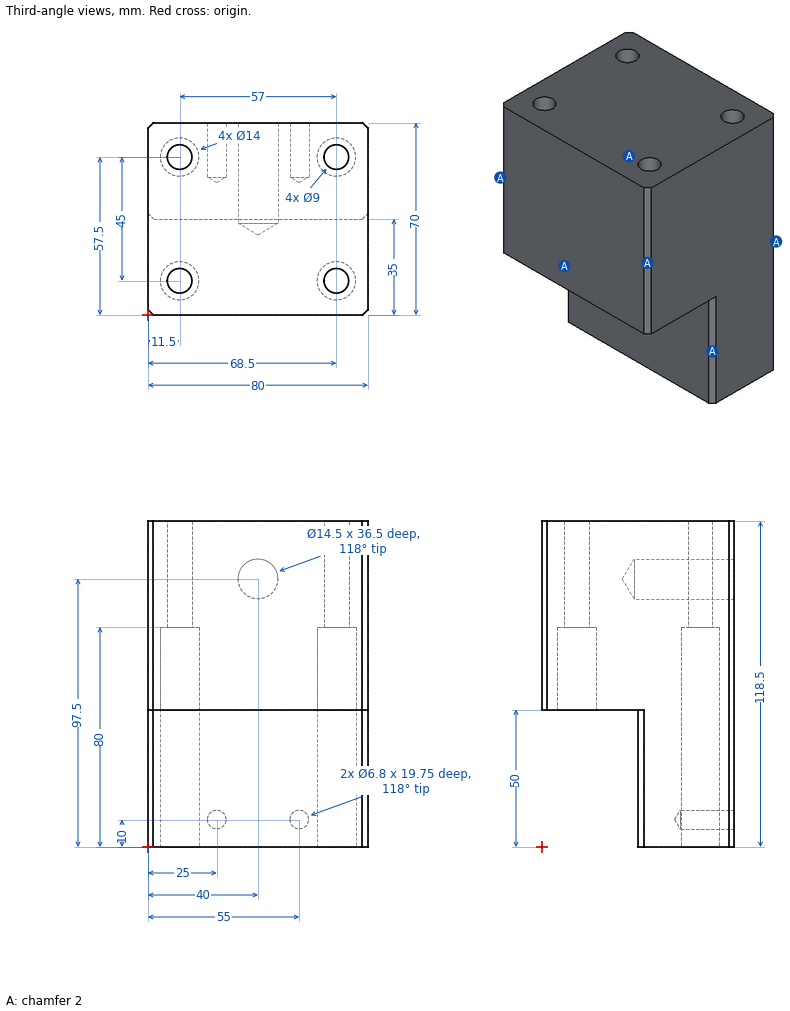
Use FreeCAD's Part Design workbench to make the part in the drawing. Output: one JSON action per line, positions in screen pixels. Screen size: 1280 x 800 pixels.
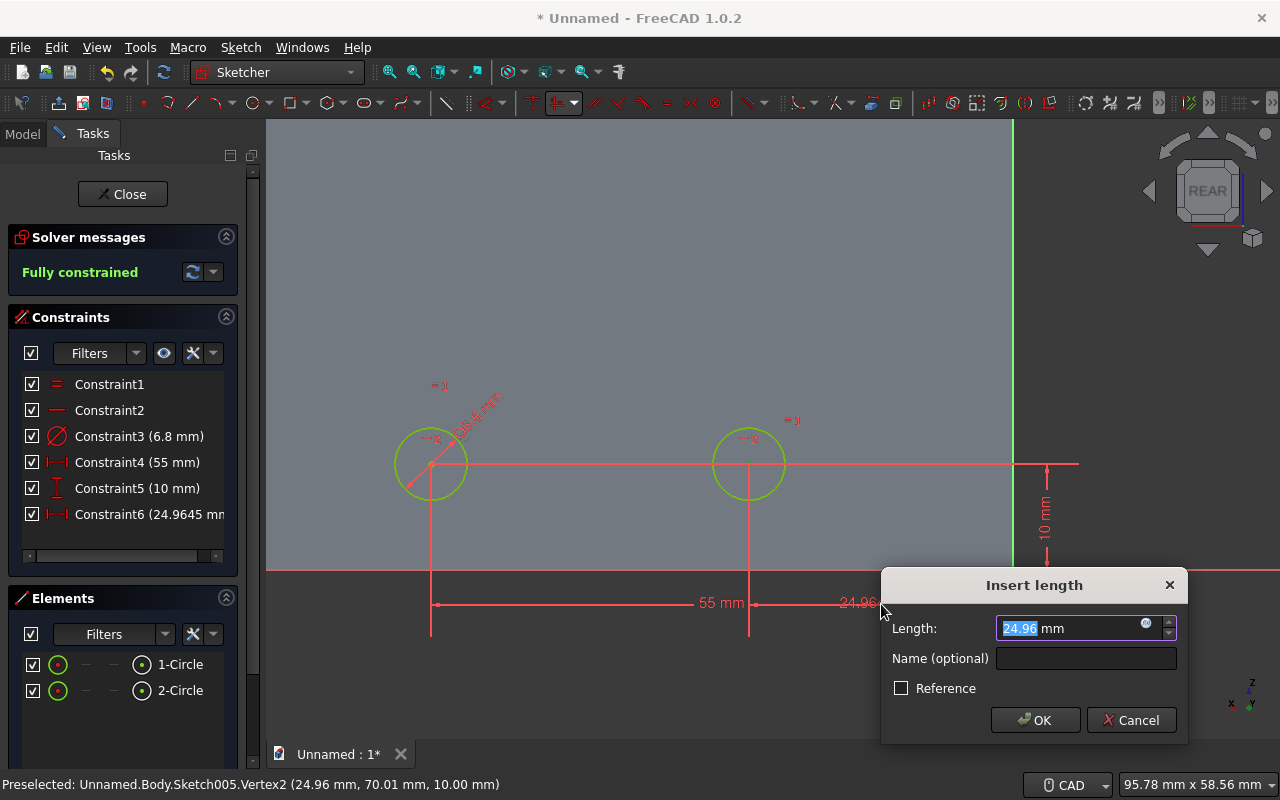
{"action": "type", "text": "25"}
{"action": "key", "text": "Return"}
{"action": "key", "text": "Escape"}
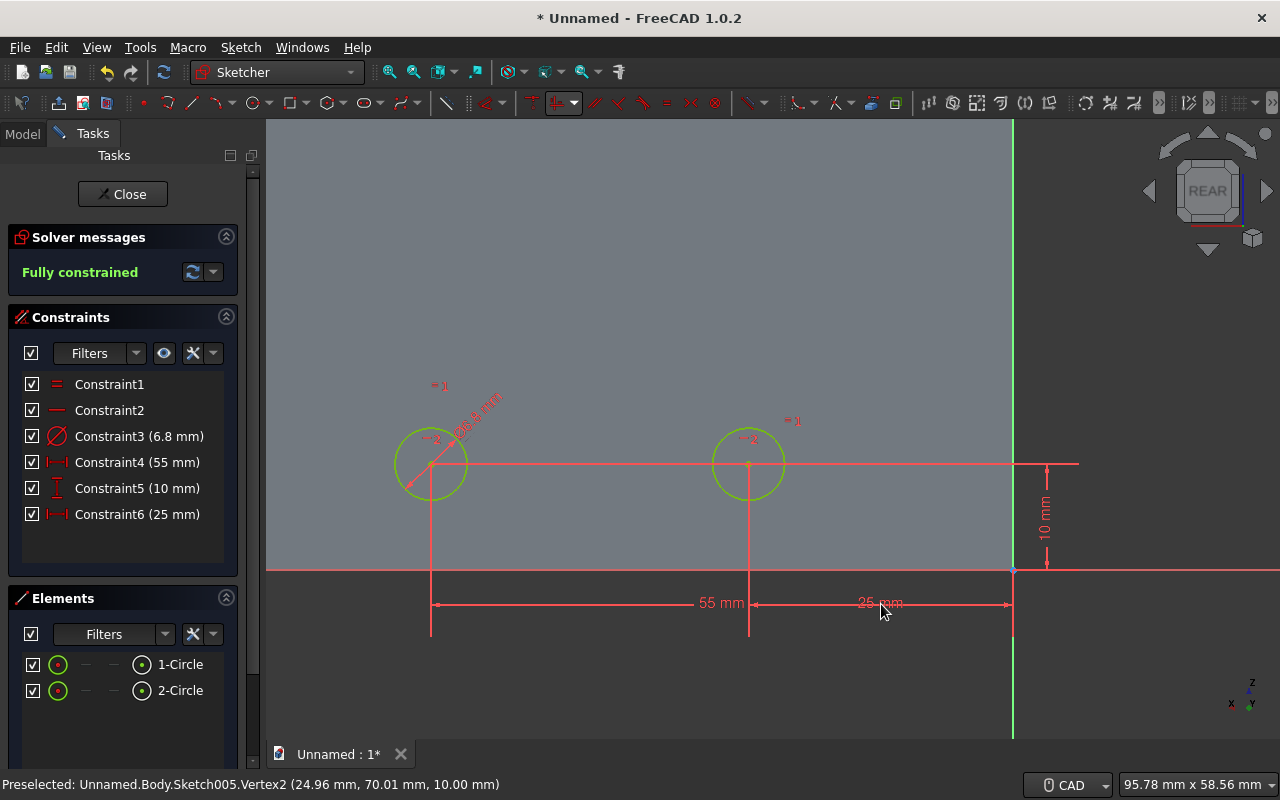
{"action": "left_click", "coordinate": [123, 194]}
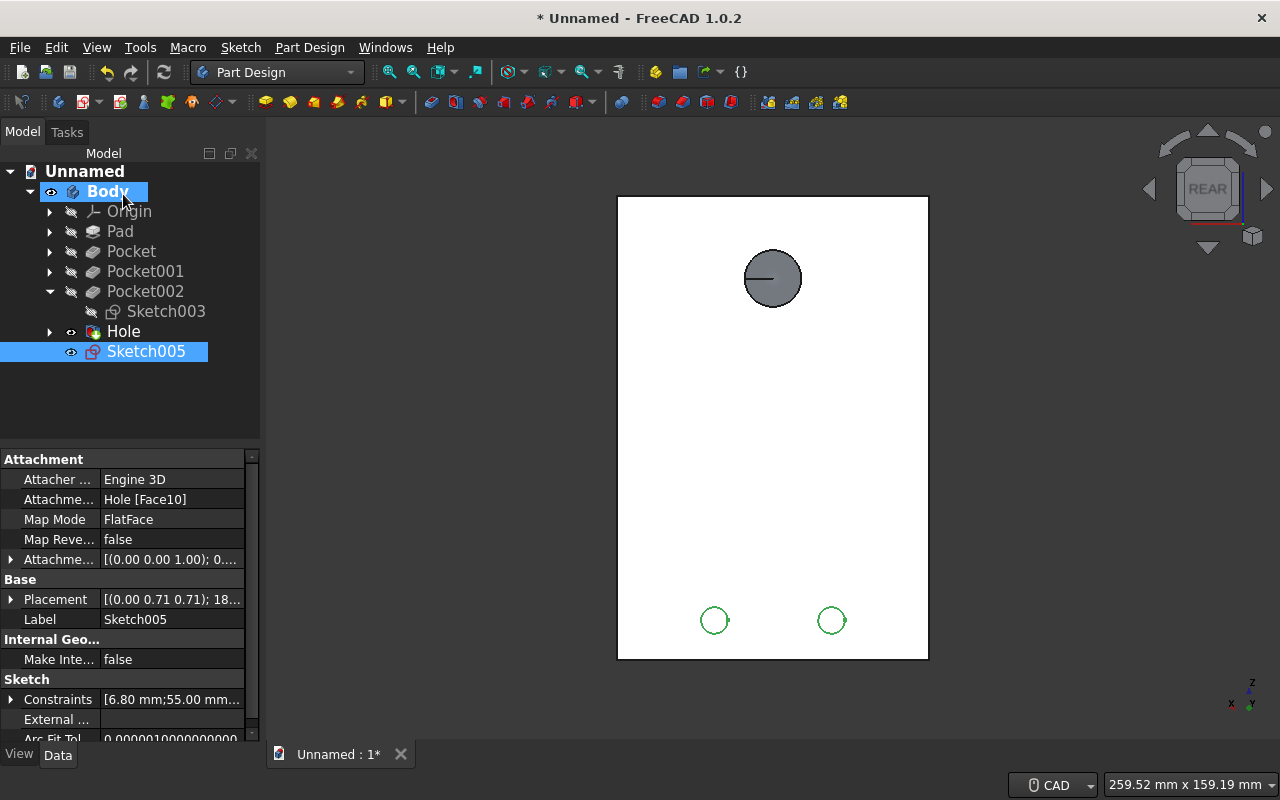
{"action": "left_click", "coordinate": [456, 102]}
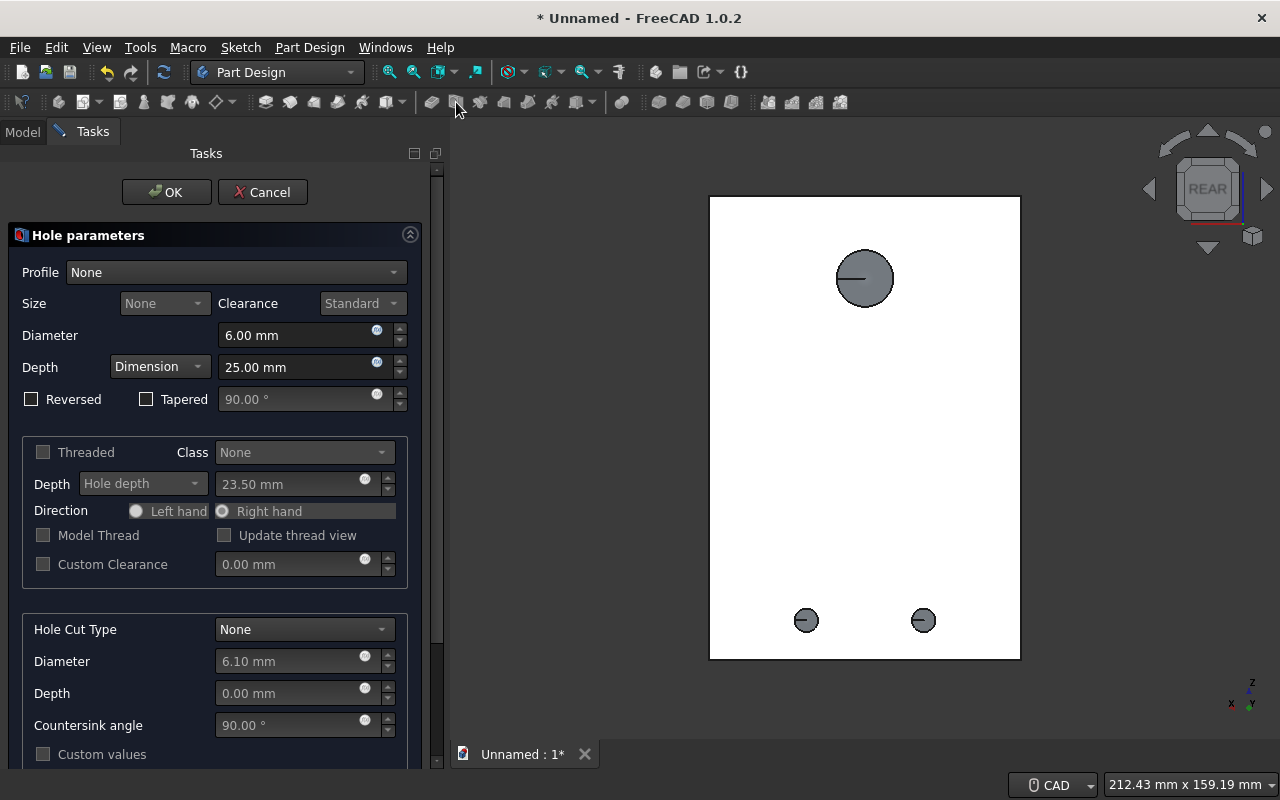
{"action": "triple_click", "coordinate": [305, 335]}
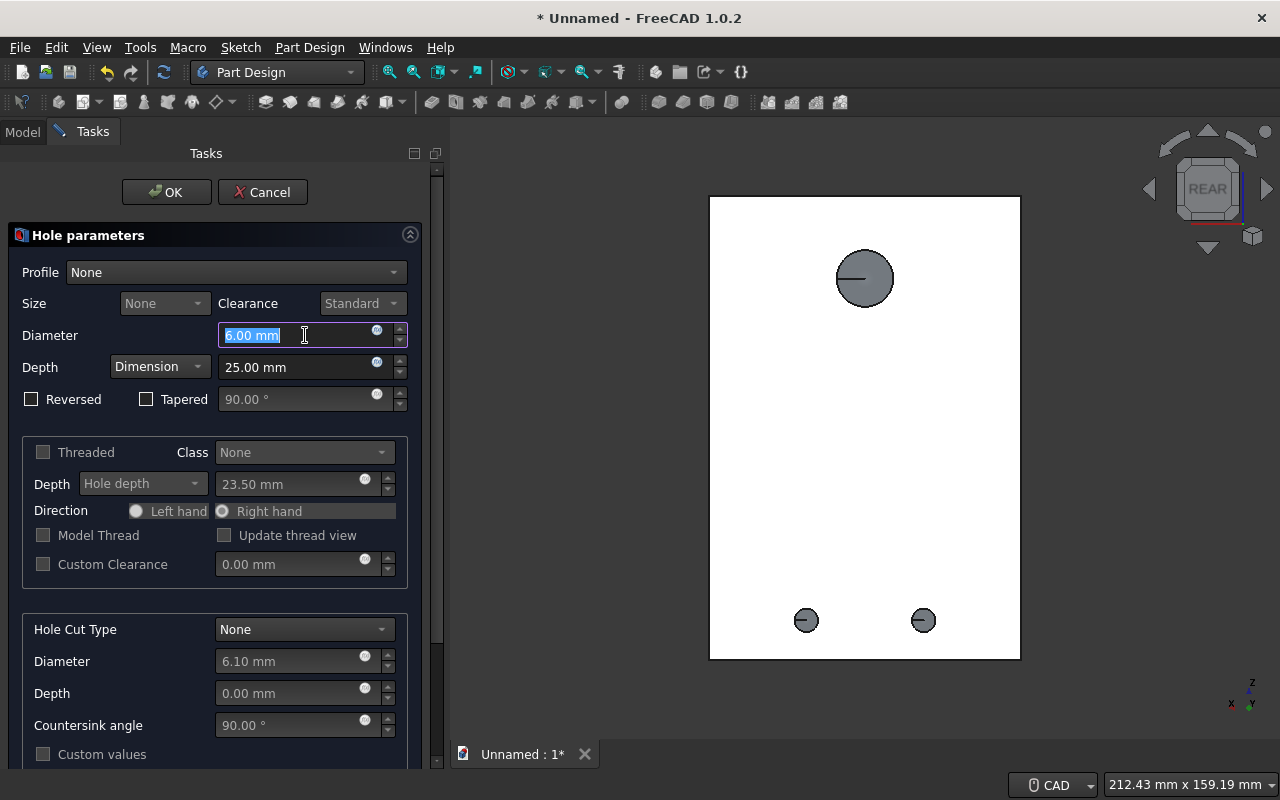
{"action": "type", "text": "6.8"}
{"action": "key", "text": "Tab"}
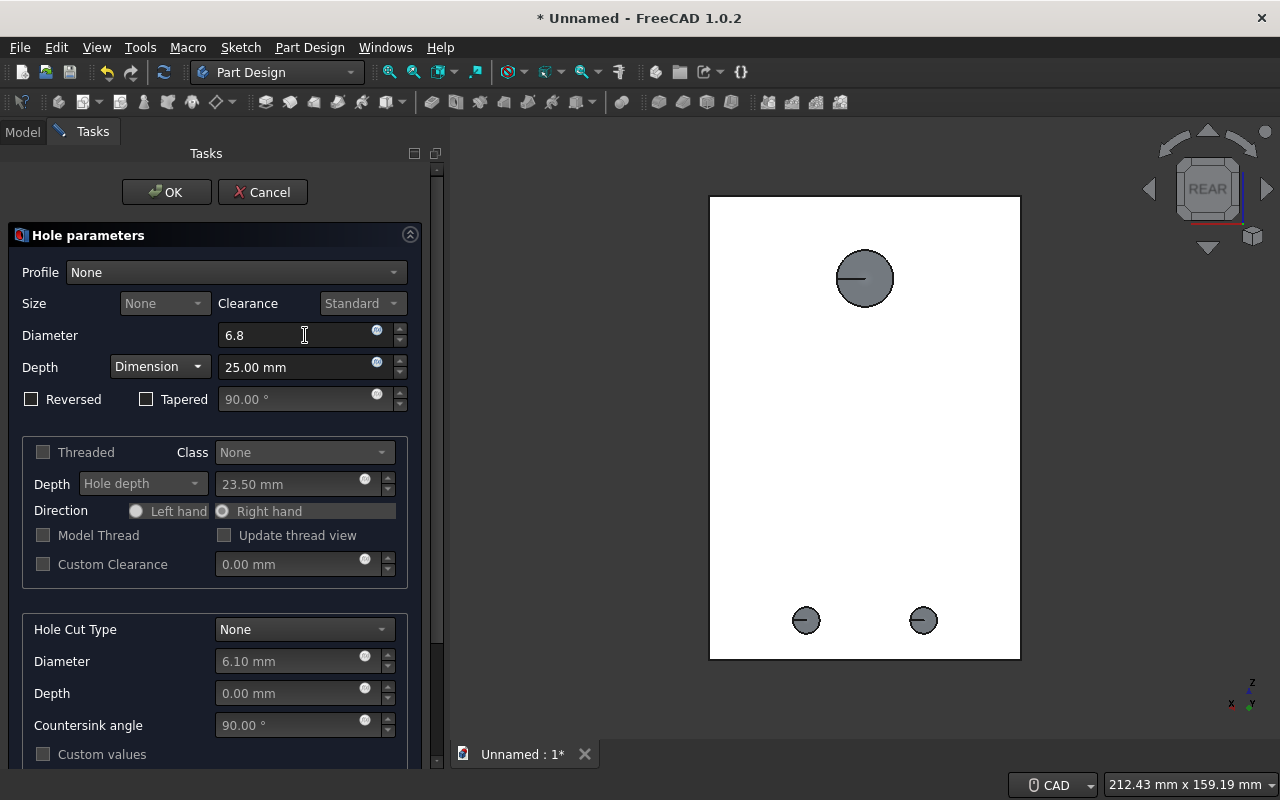
{"action": "triple_click", "coordinate": [305, 367]}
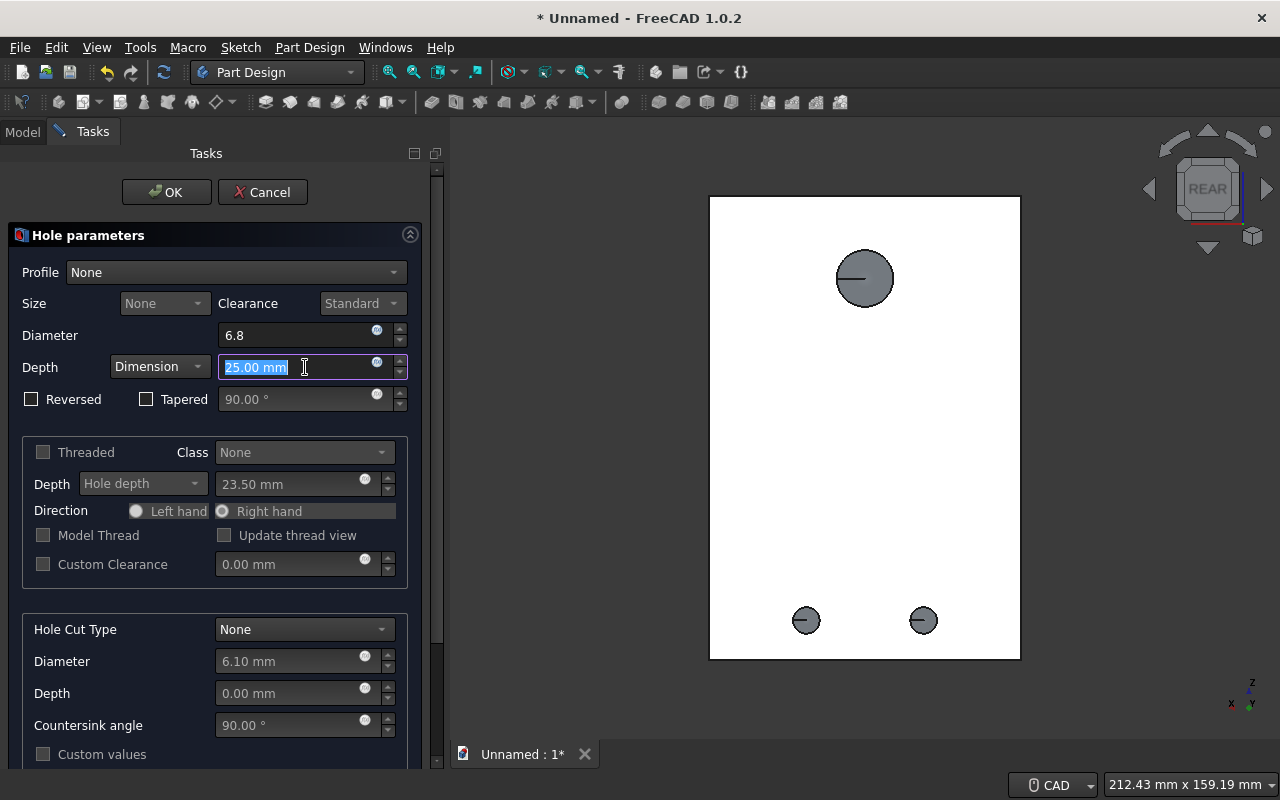
{"action": "type", "text": "19.75"}
{"action": "key", "text": "Tab"}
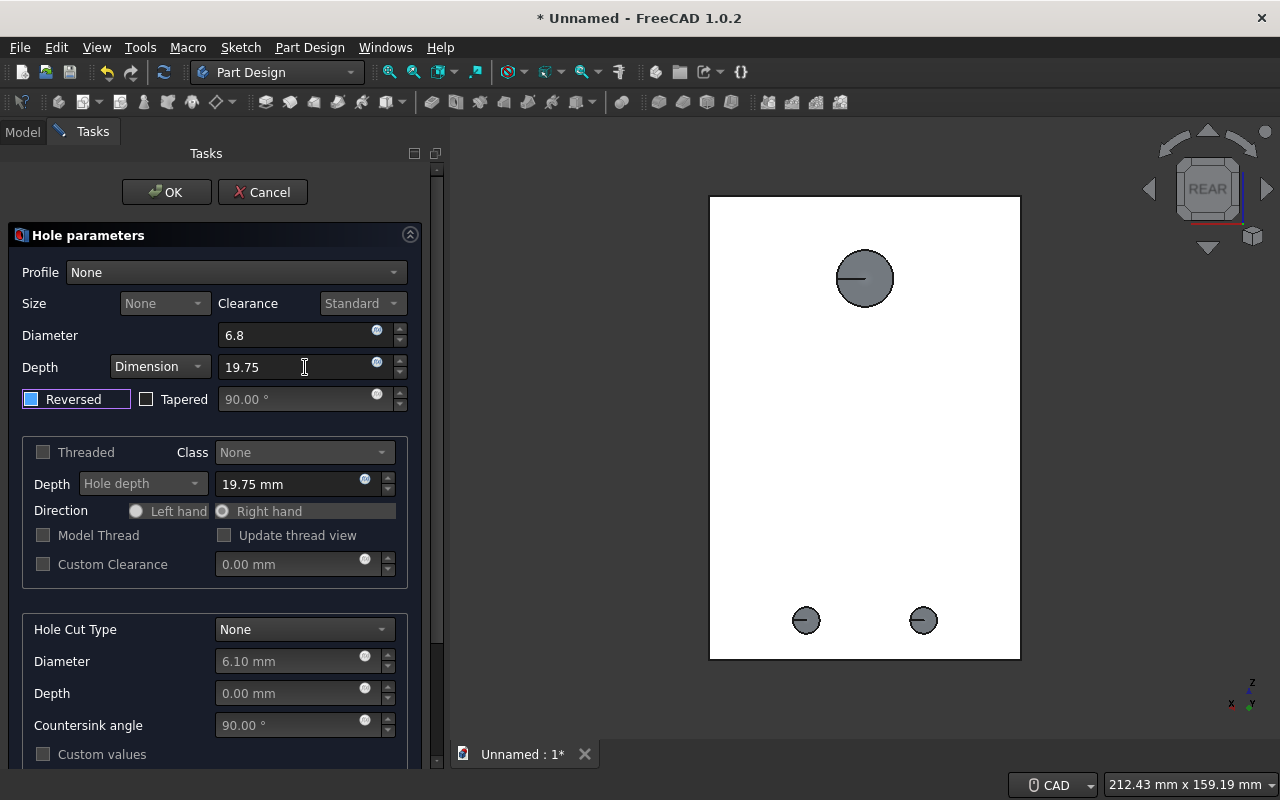
{"action": "left_click", "coordinate": [167, 192]}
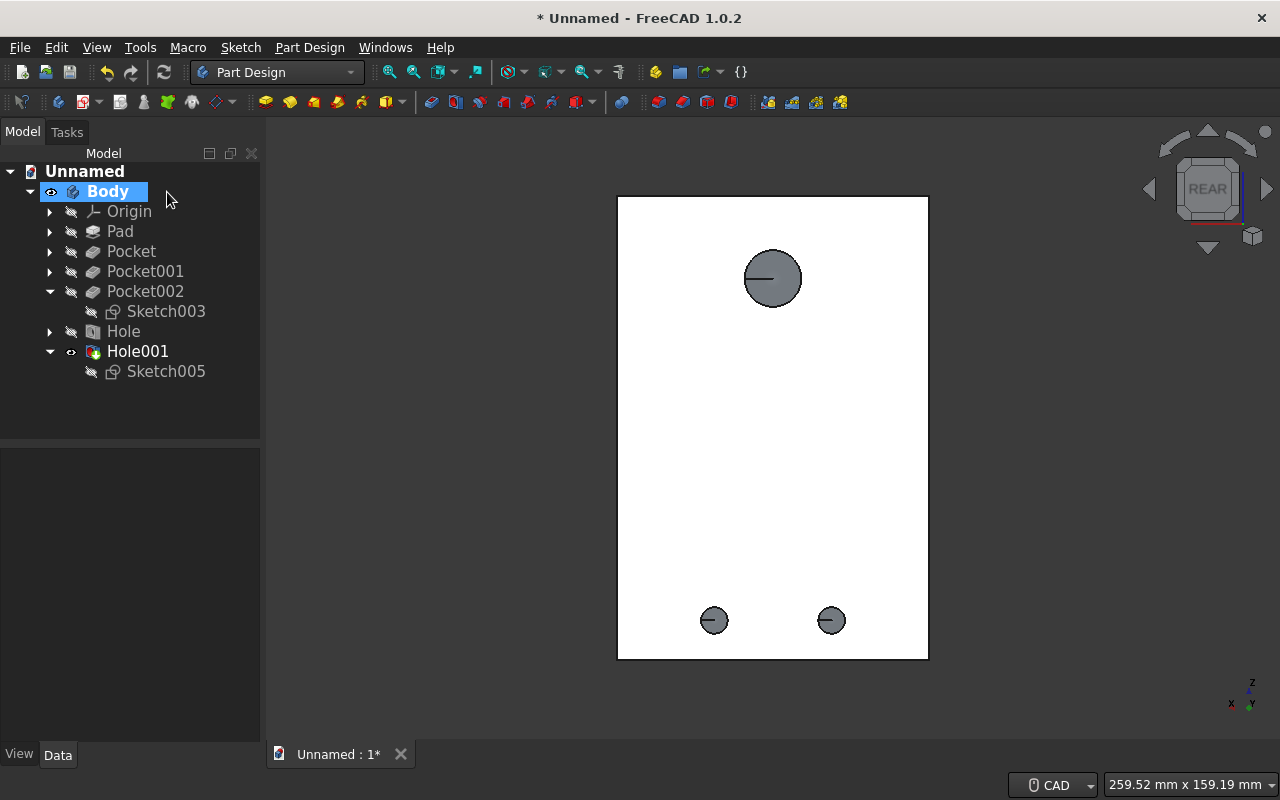
{"action": "left_click", "coordinate": [929, 427]}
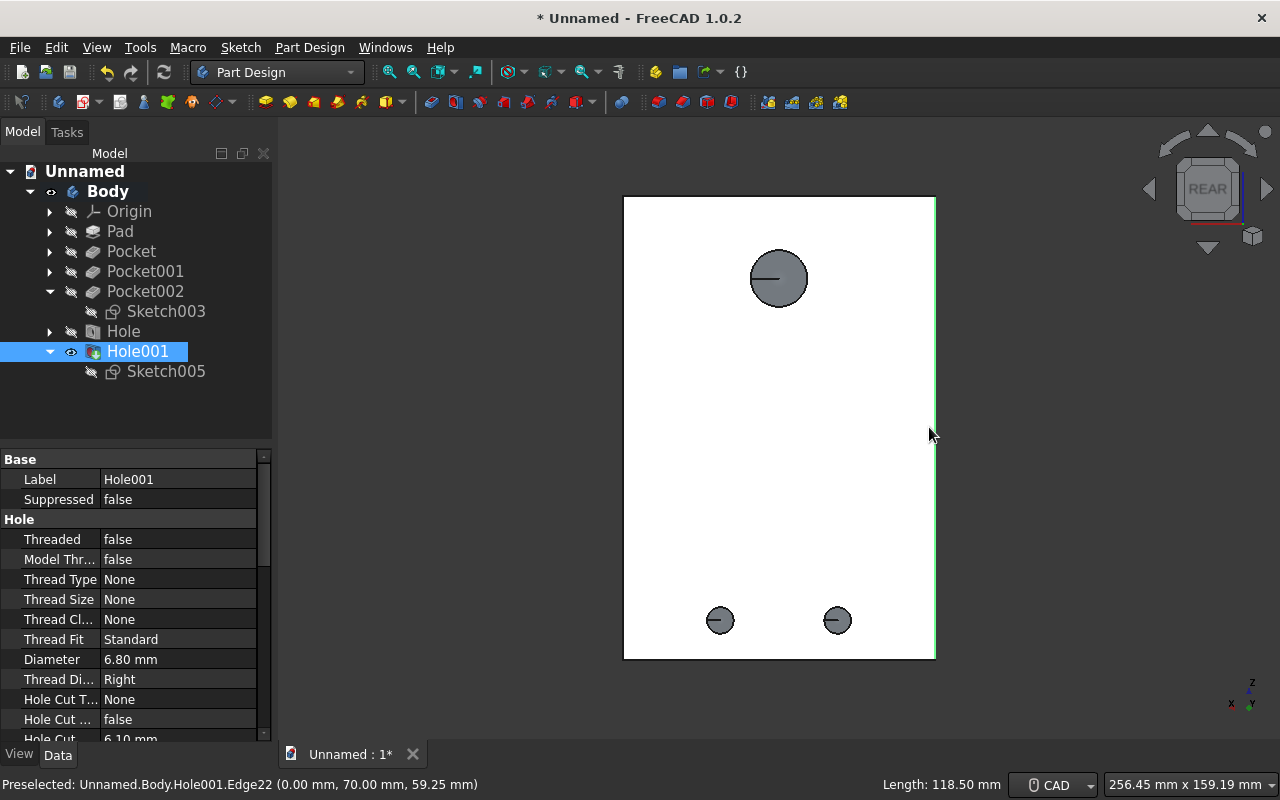
{"action": "key", "text": "0"}